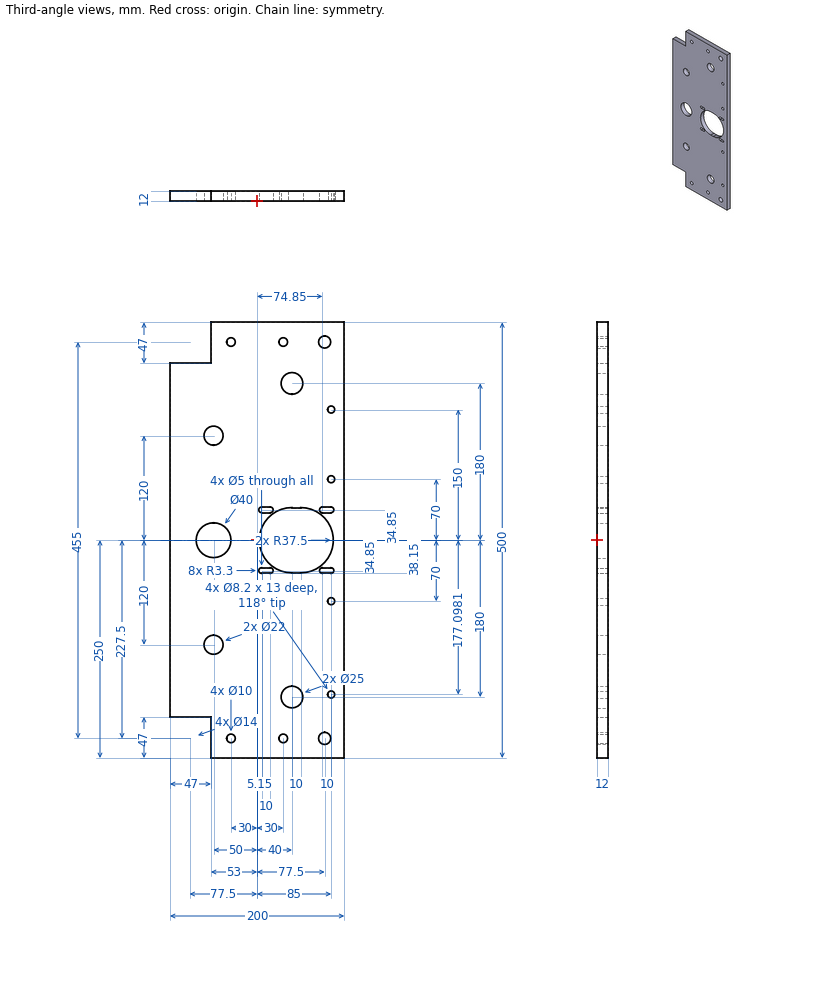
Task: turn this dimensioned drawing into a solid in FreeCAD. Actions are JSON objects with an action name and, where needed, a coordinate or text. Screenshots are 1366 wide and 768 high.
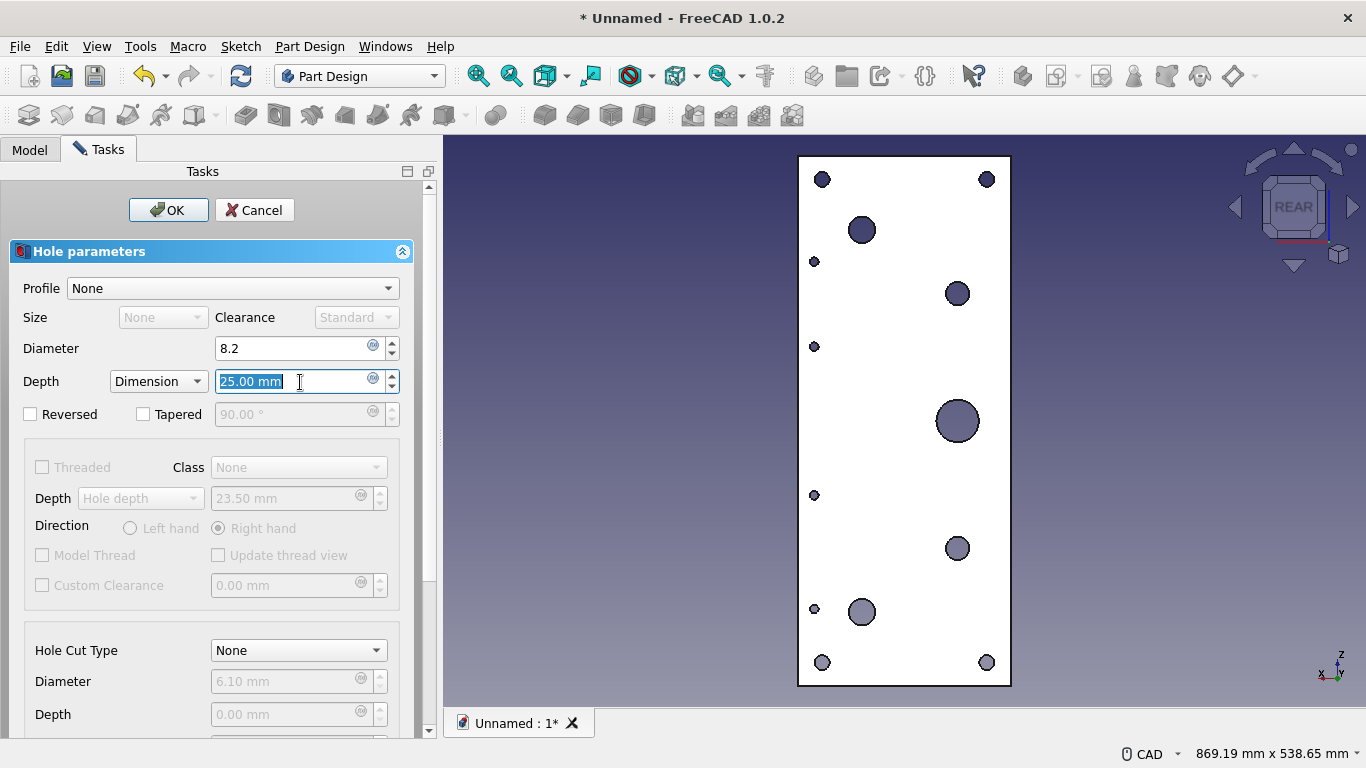
{"action": "type", "text": "13"}
{"action": "key", "text": "Tab"}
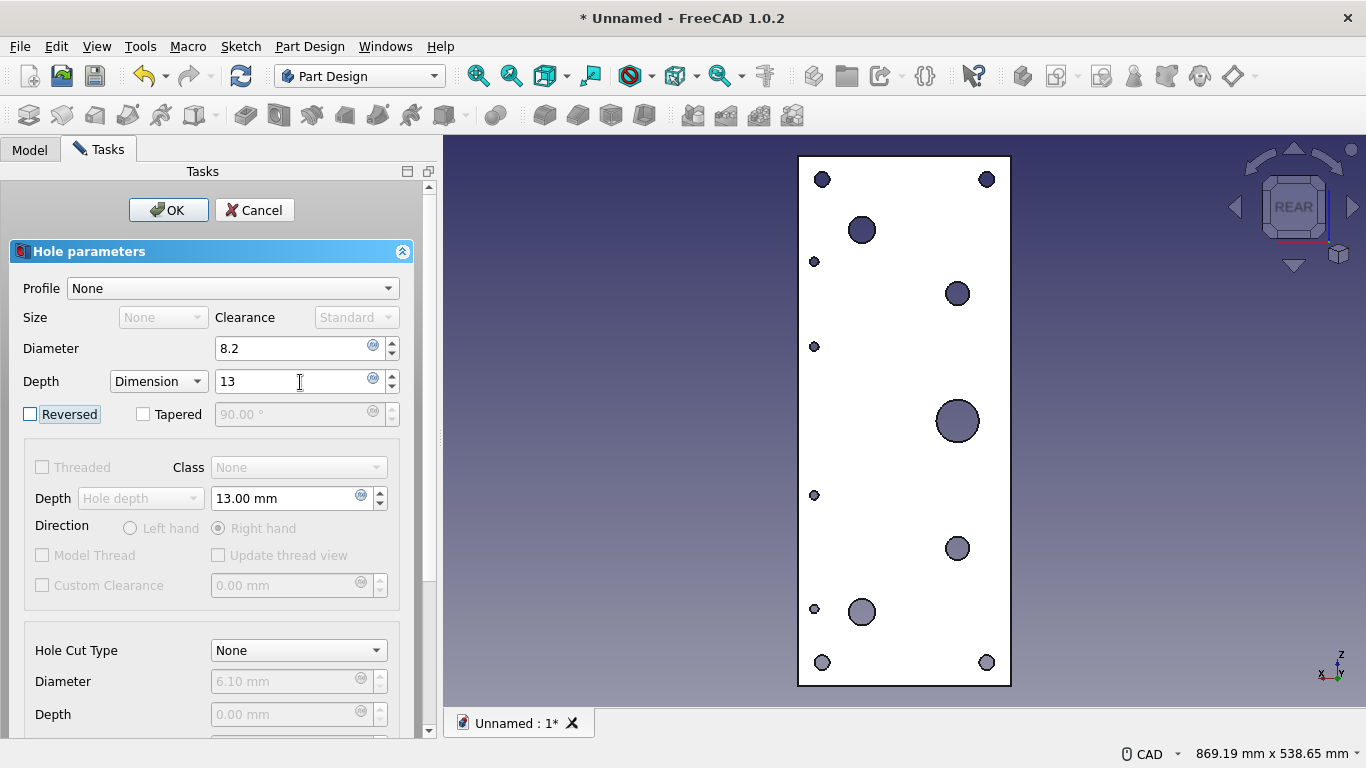
{"action": "left_click", "coordinate": [169, 210]}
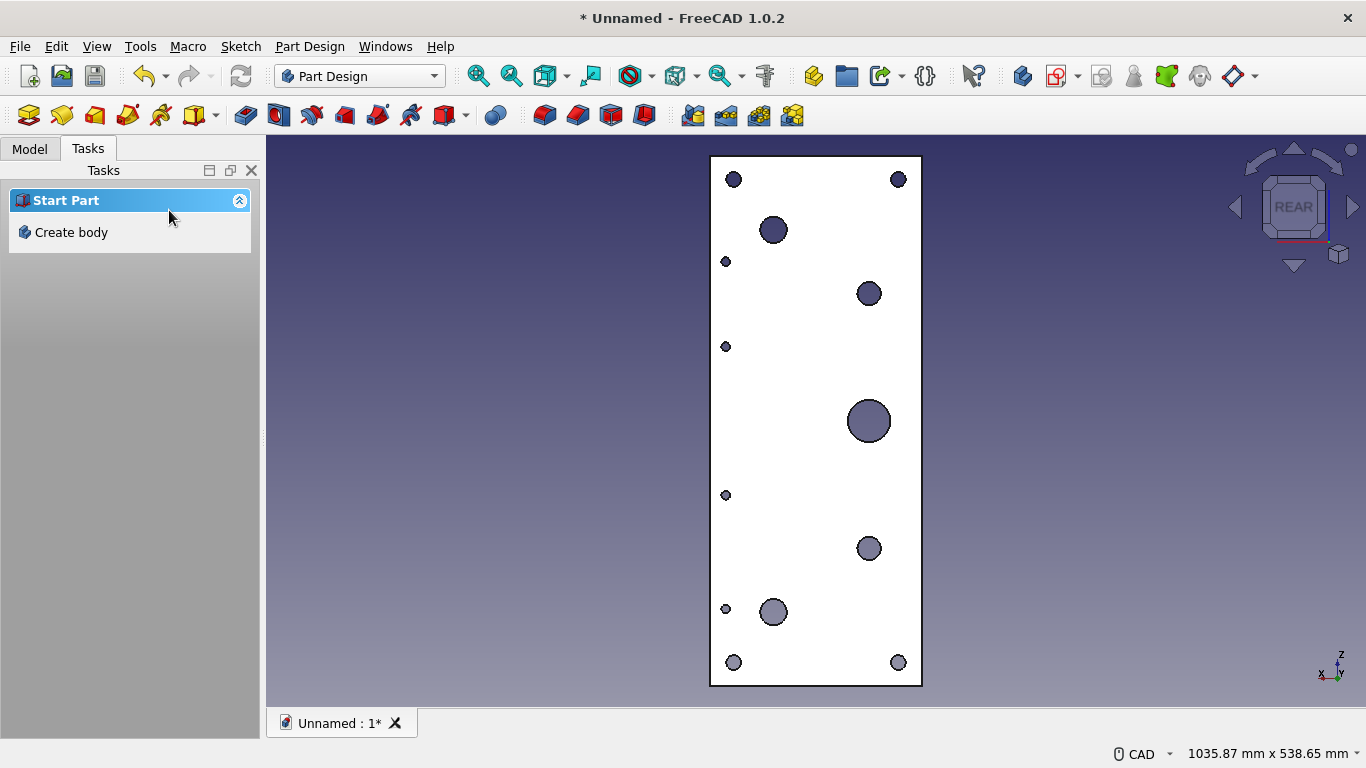
{"action": "left_click", "coordinate": [816, 496]}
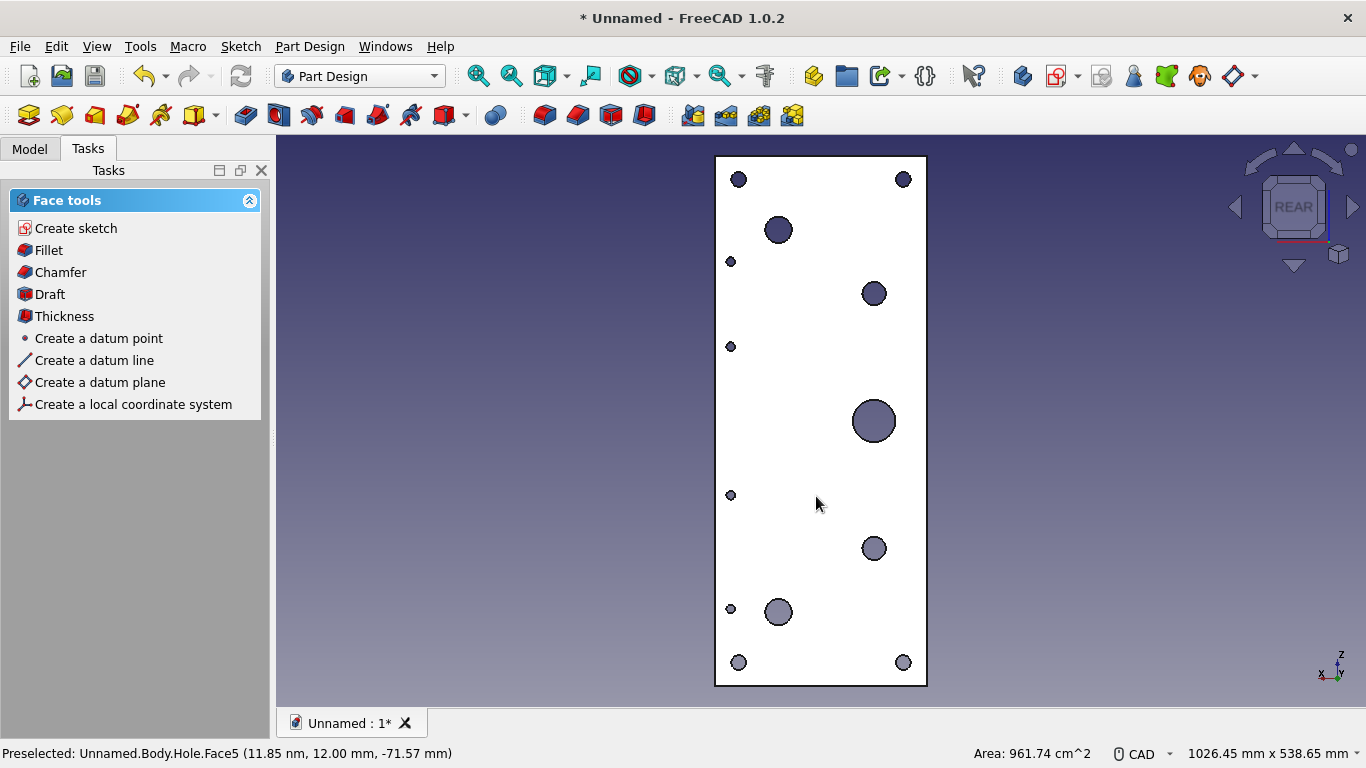
{"action": "left_click", "coordinate": [1056, 76]}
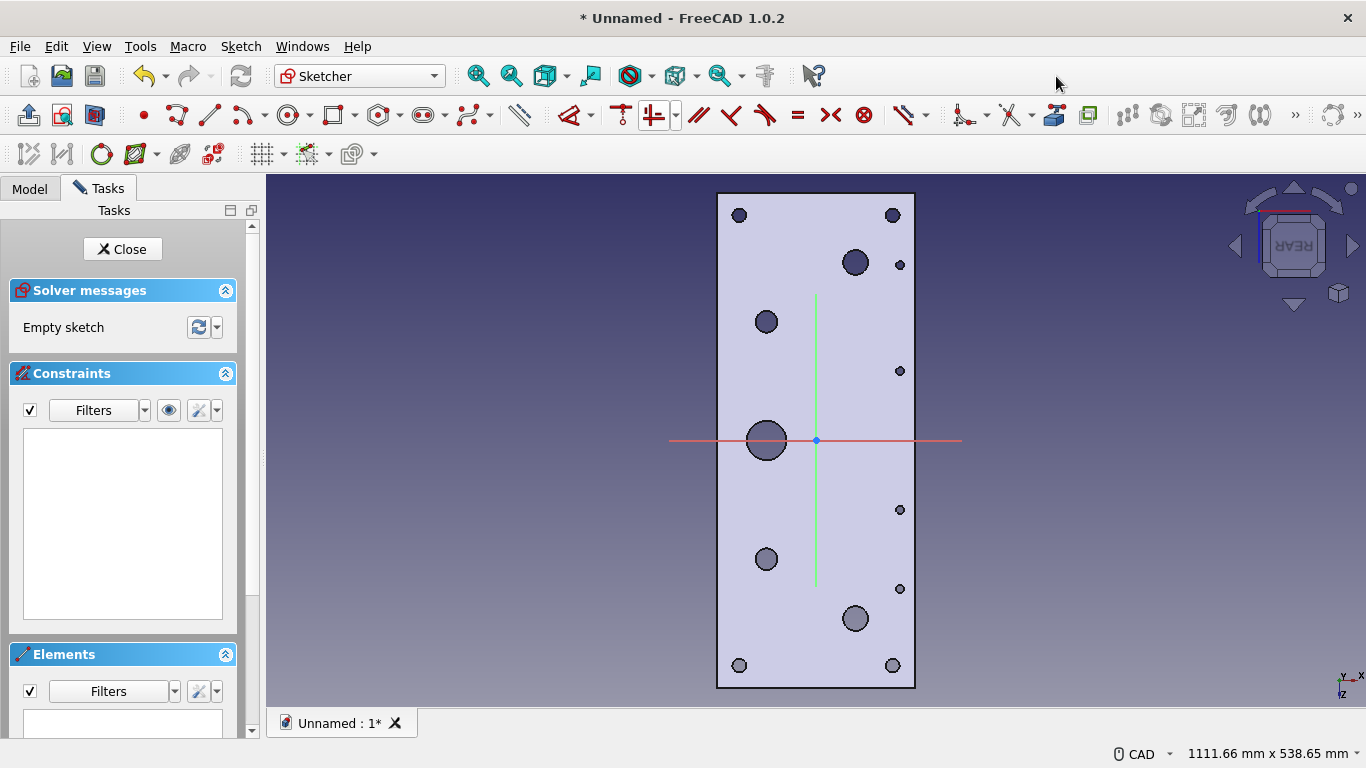
{"action": "scroll", "coordinate": [608, 441], "scroll_direction": "down", "scroll_amount": 2}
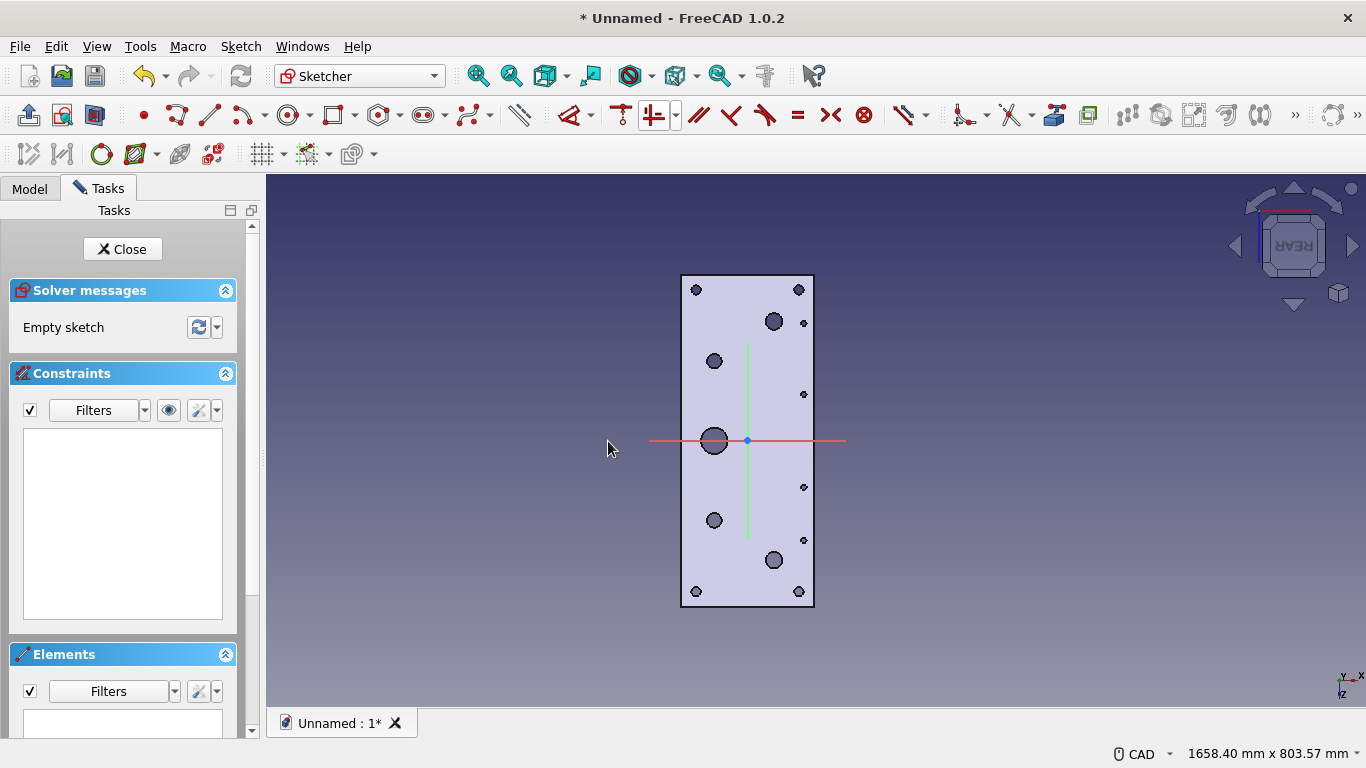
{"action": "key", "text": "g c"}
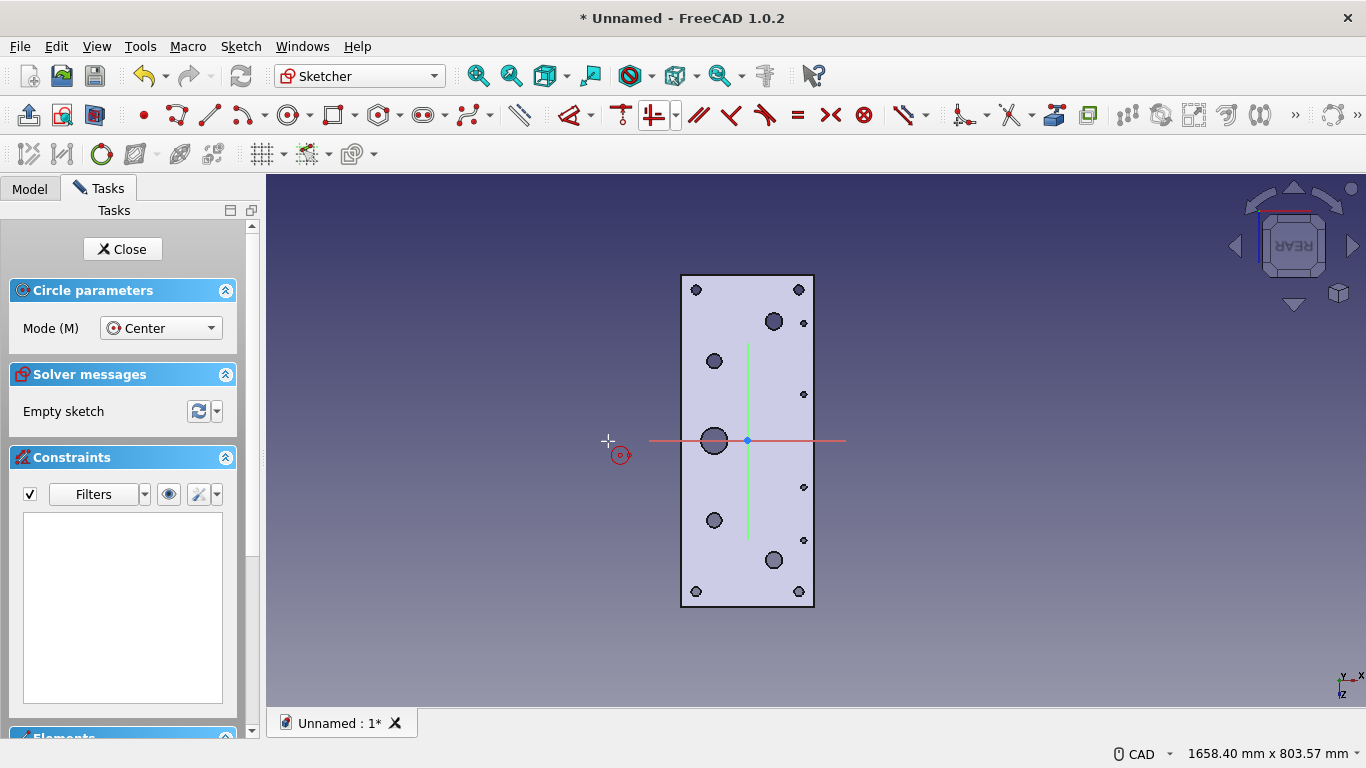
{"action": "scroll", "coordinate": [728, 290], "scroll_direction": "up", "scroll_amount": 10}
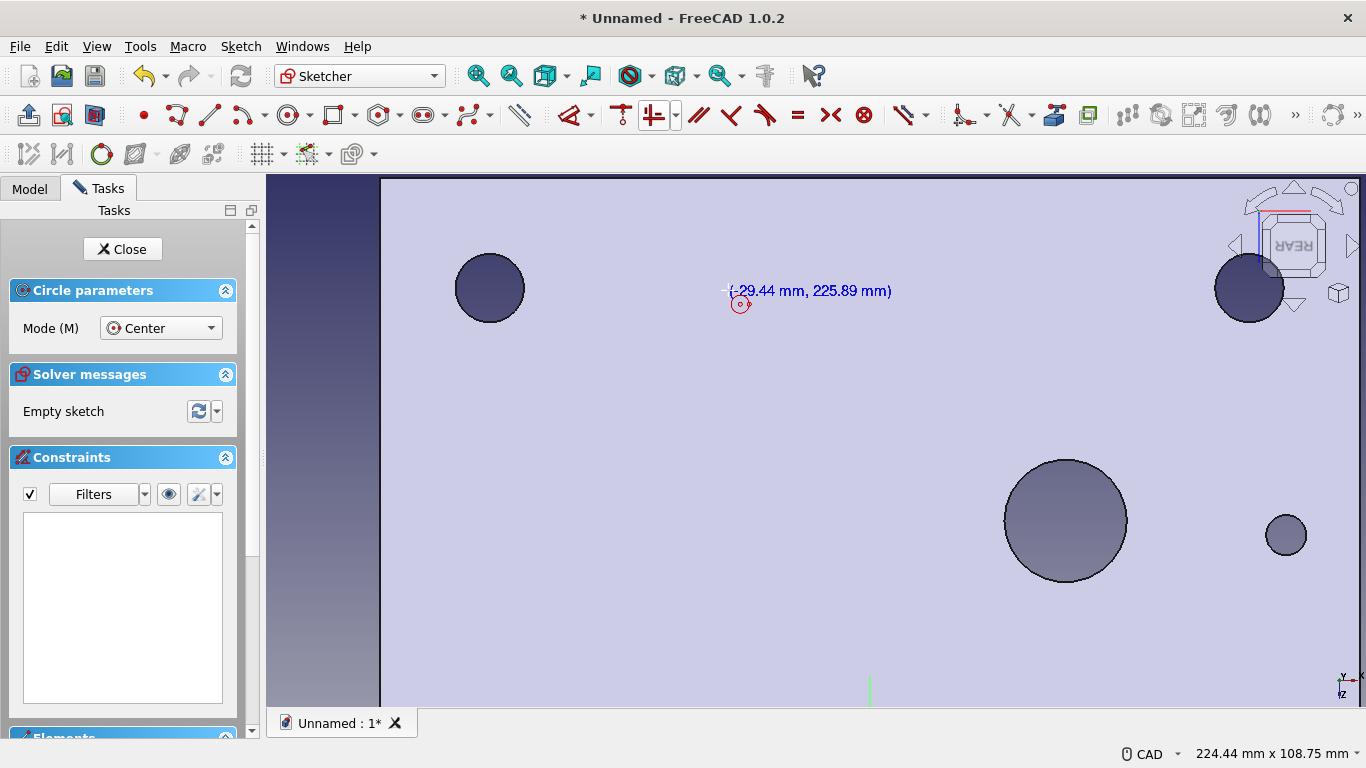
{"action": "scroll", "coordinate": [728, 290], "scroll_direction": "down", "scroll_amount": 10}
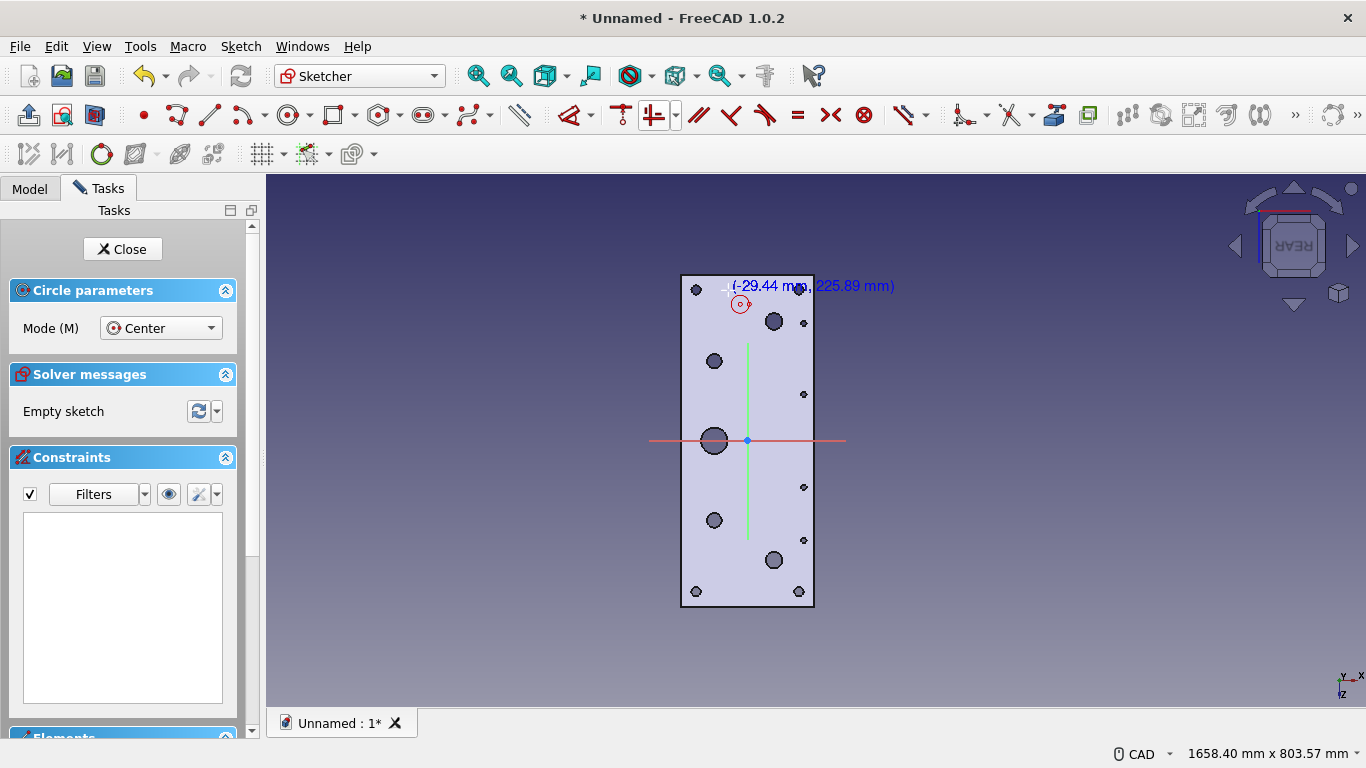
{"action": "left_click", "coordinate": [728, 290]}
{"action": "mouse_move", "coordinate": [730, 288]}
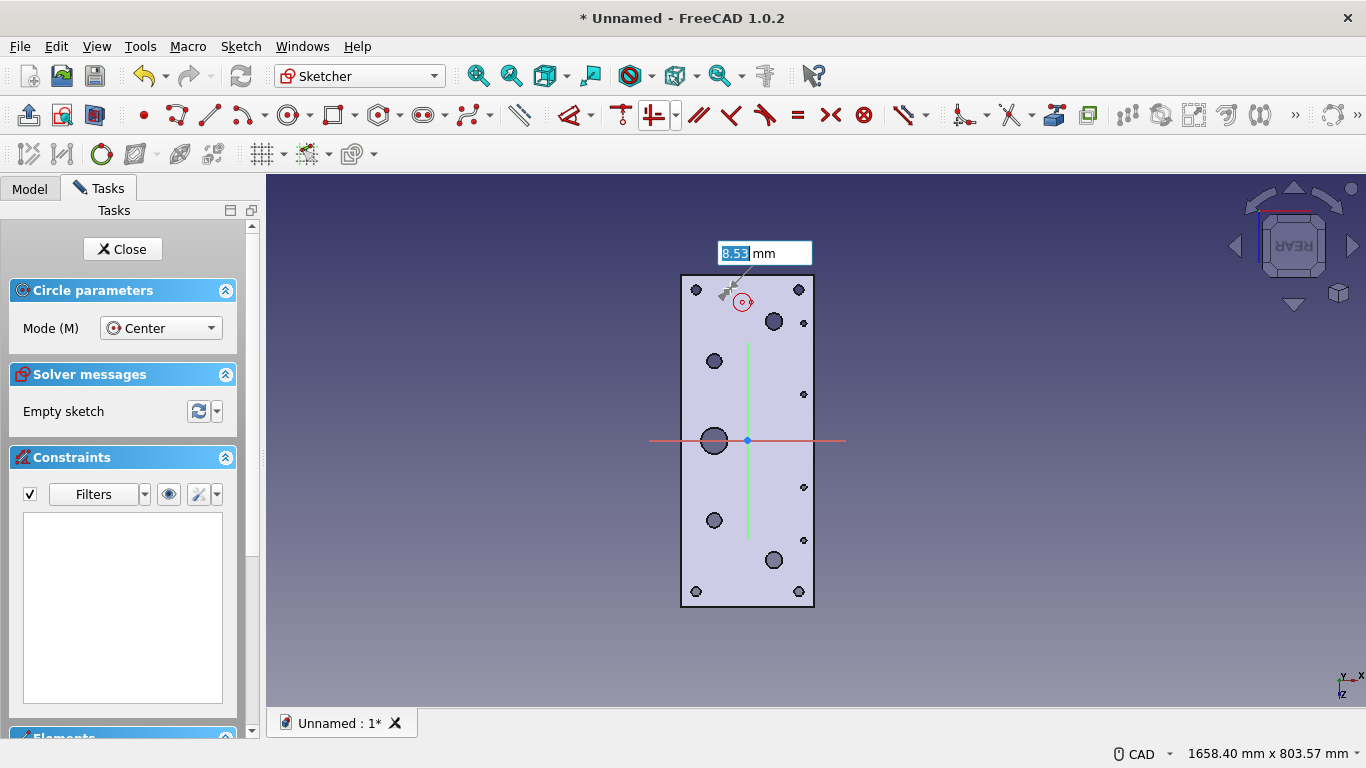
{"action": "type", "text": "10"}
{"action": "key", "text": "Return"}